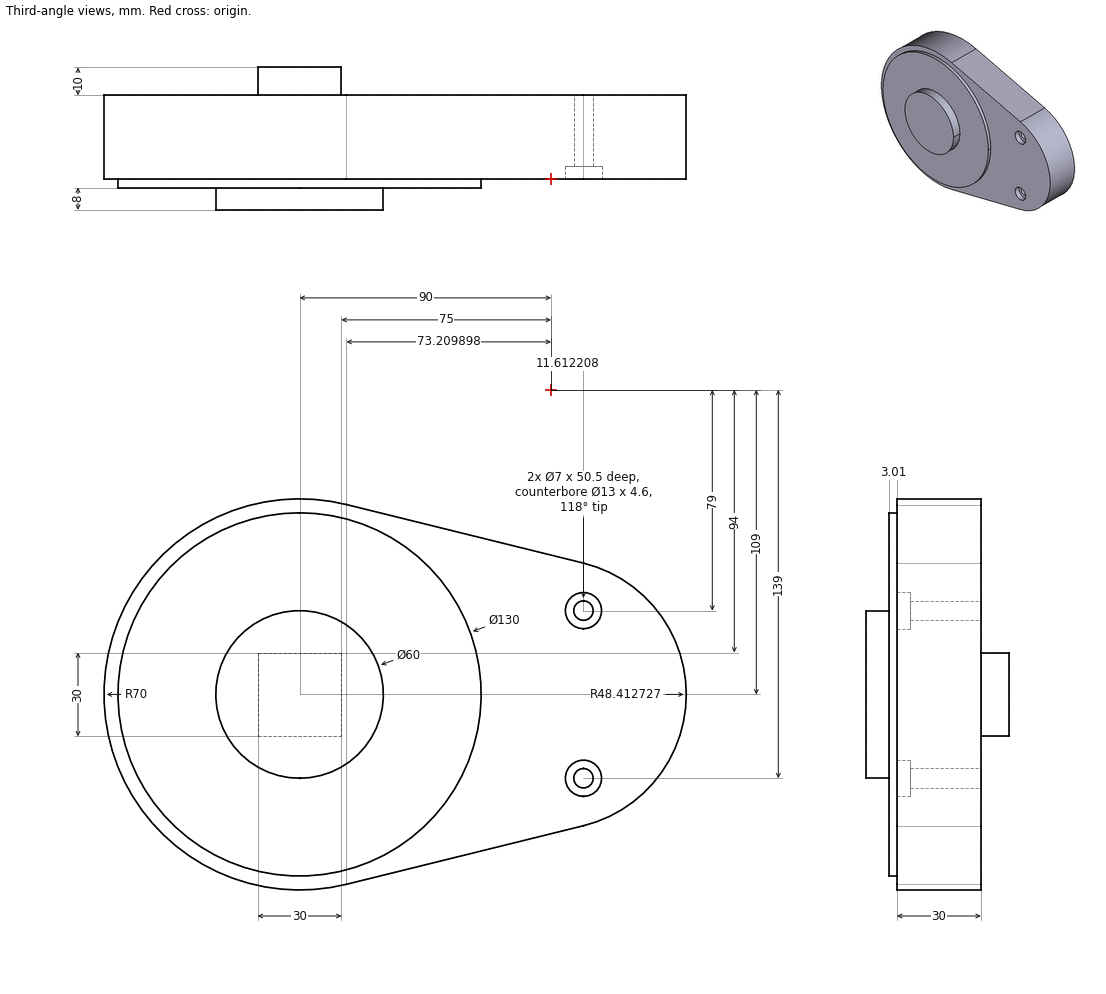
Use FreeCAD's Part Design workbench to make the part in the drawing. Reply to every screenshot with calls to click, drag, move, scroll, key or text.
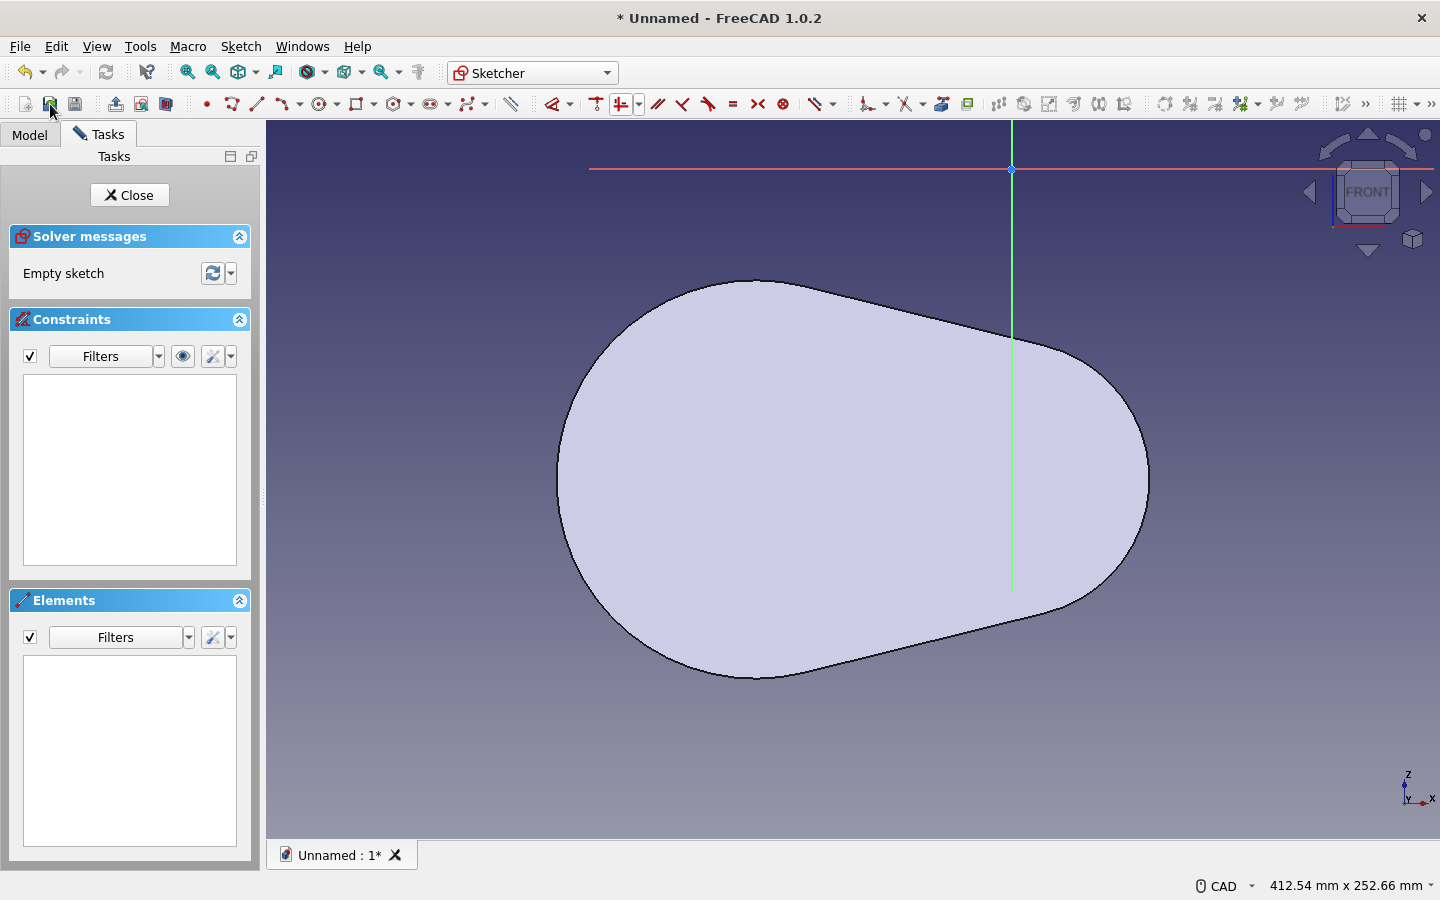
scroll(754, 762, down, 1)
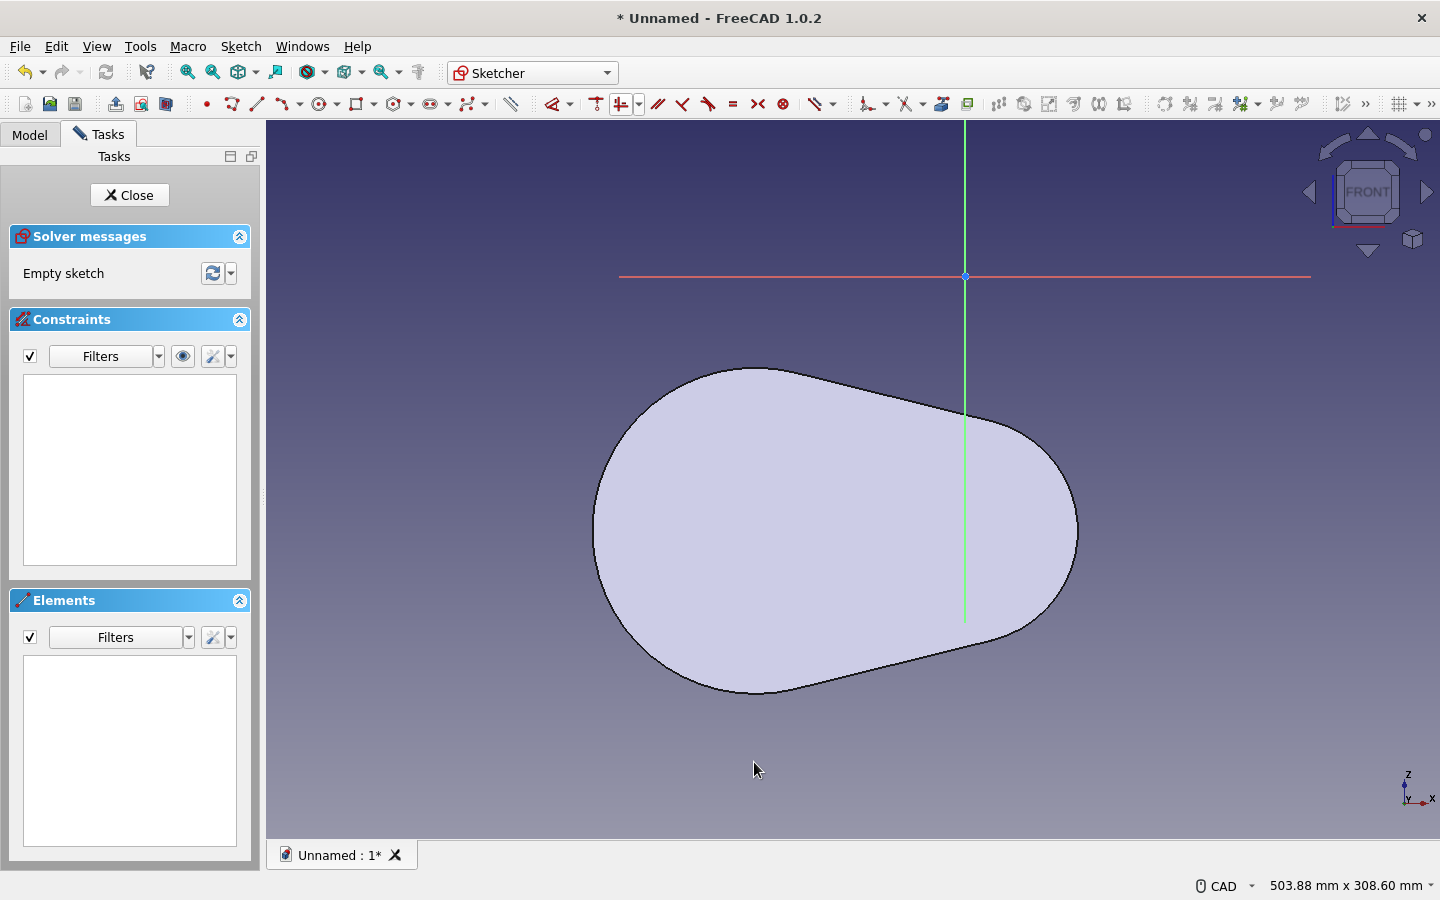
key(g)
key(c)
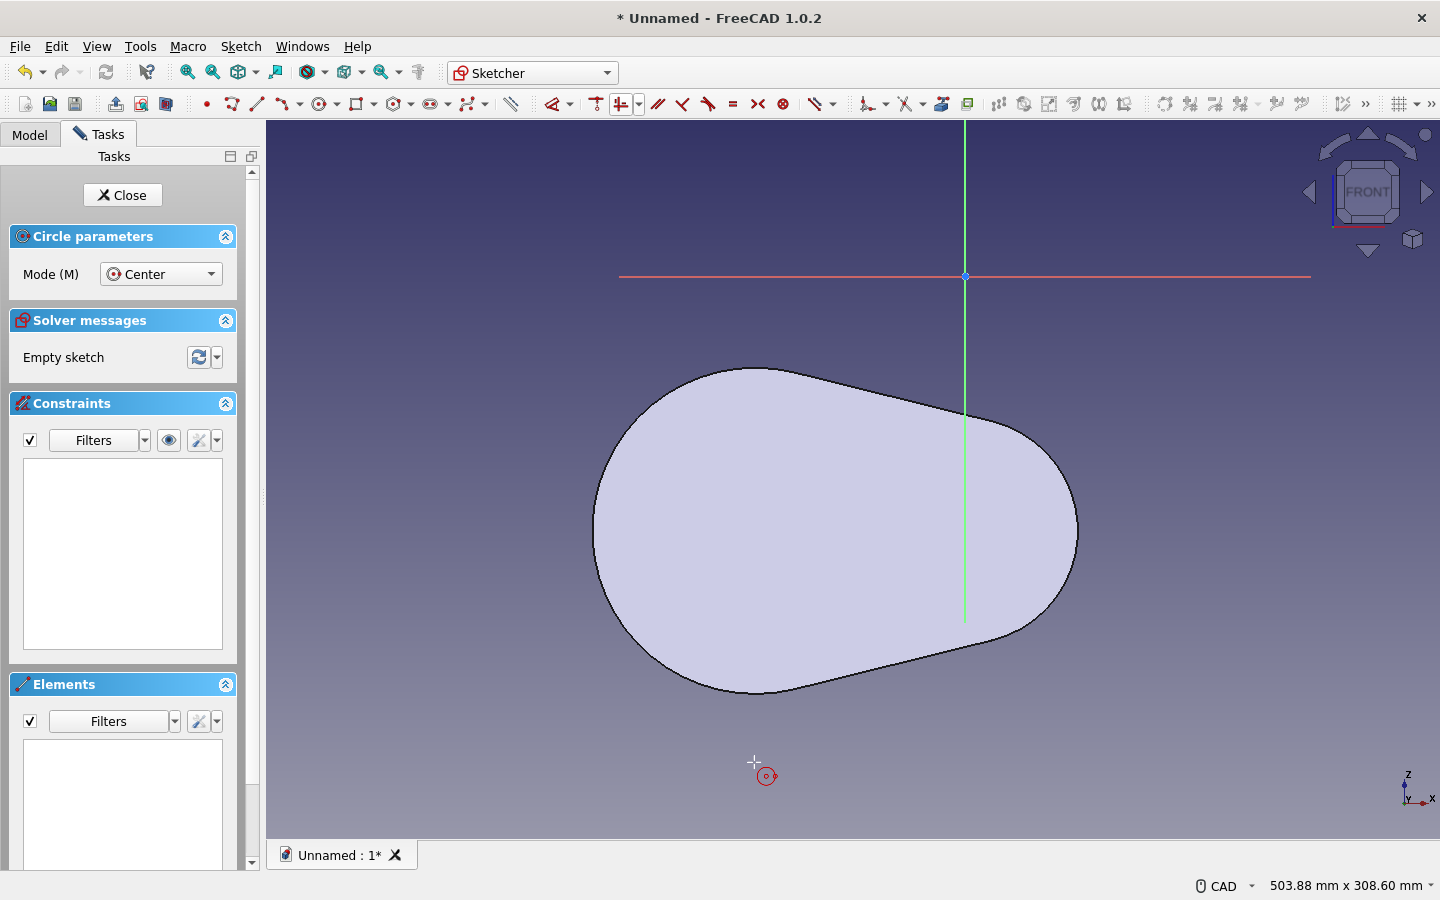
click(755, 531)
click(863, 424)
key(Escape)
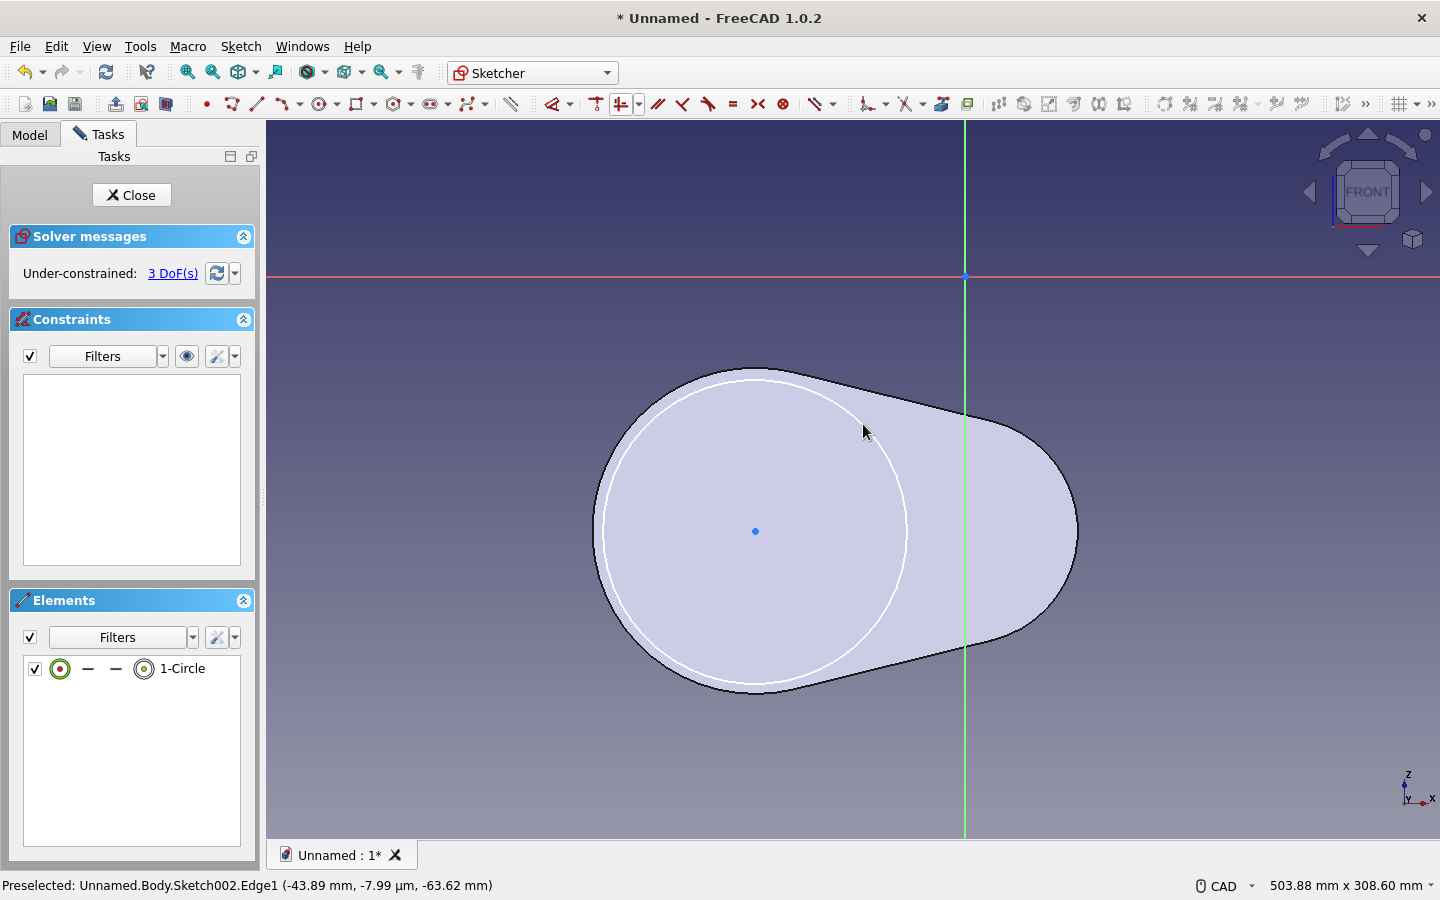
key(d)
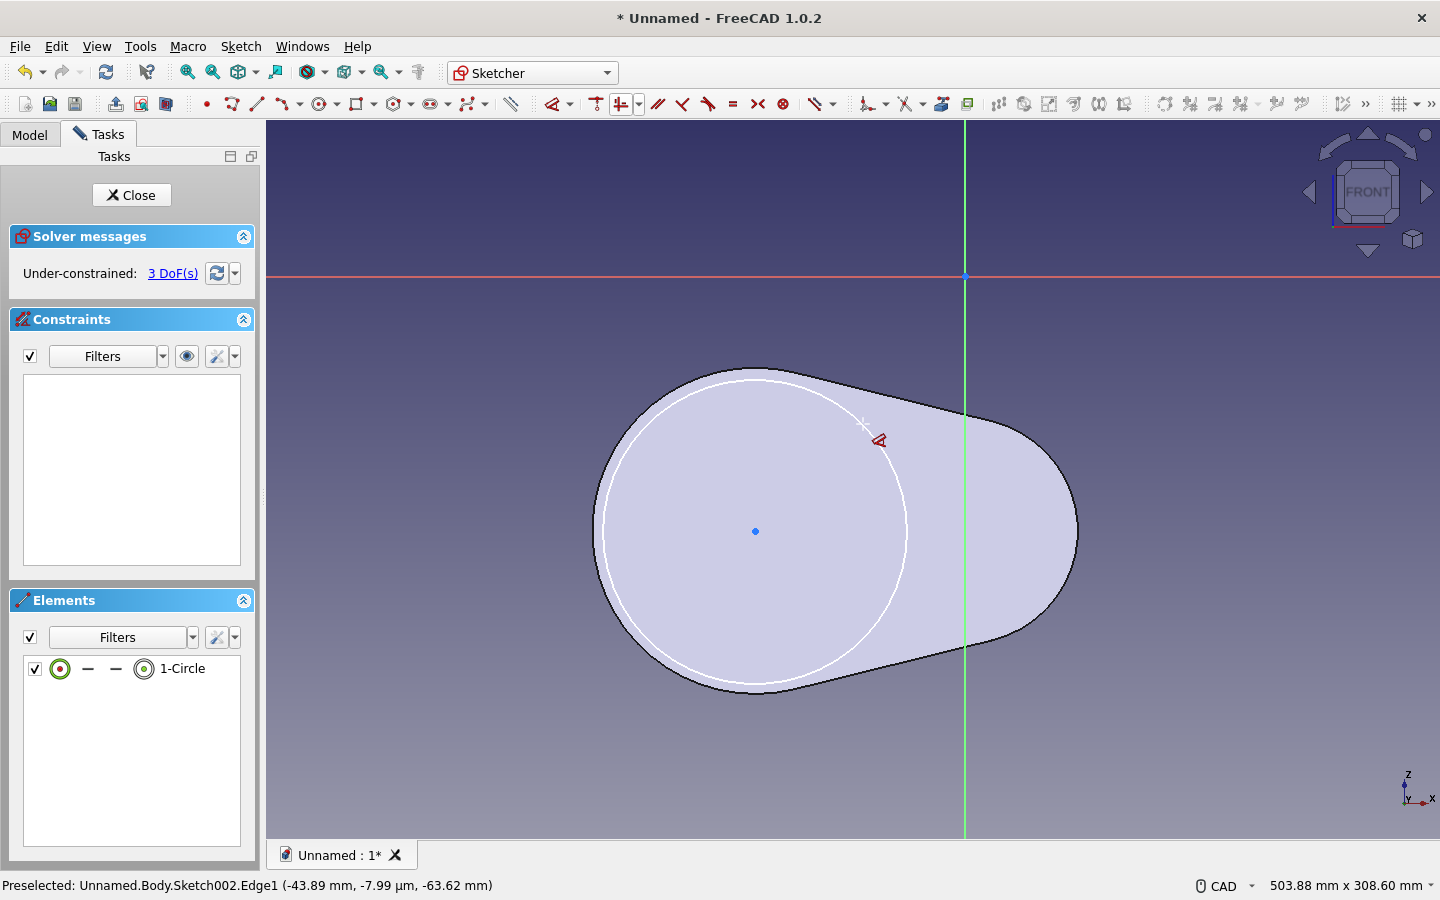
click(862, 424)
click(885, 401)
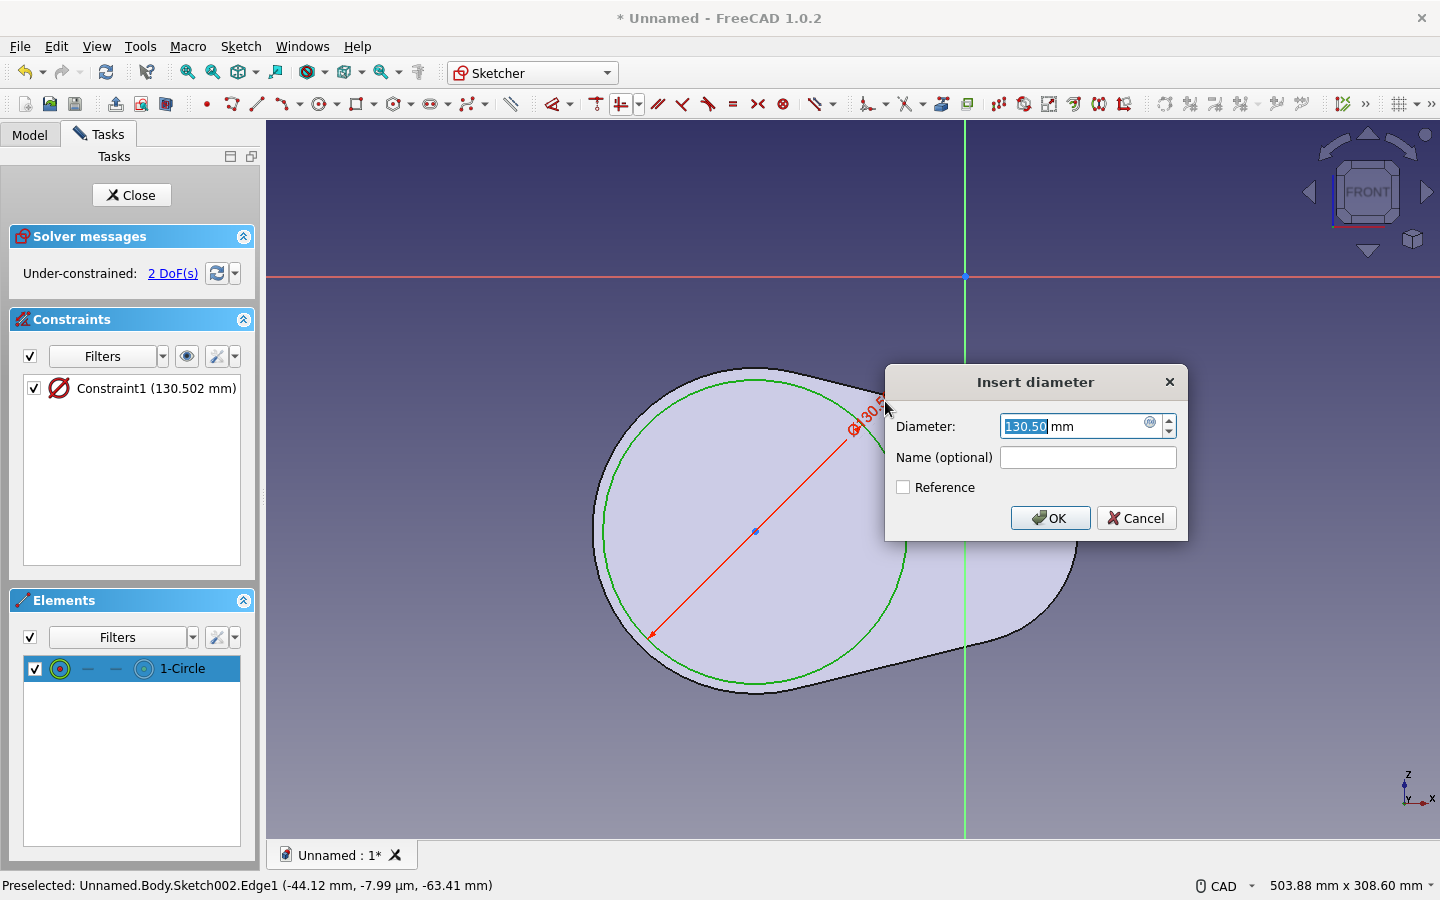
text(130)
key(Return)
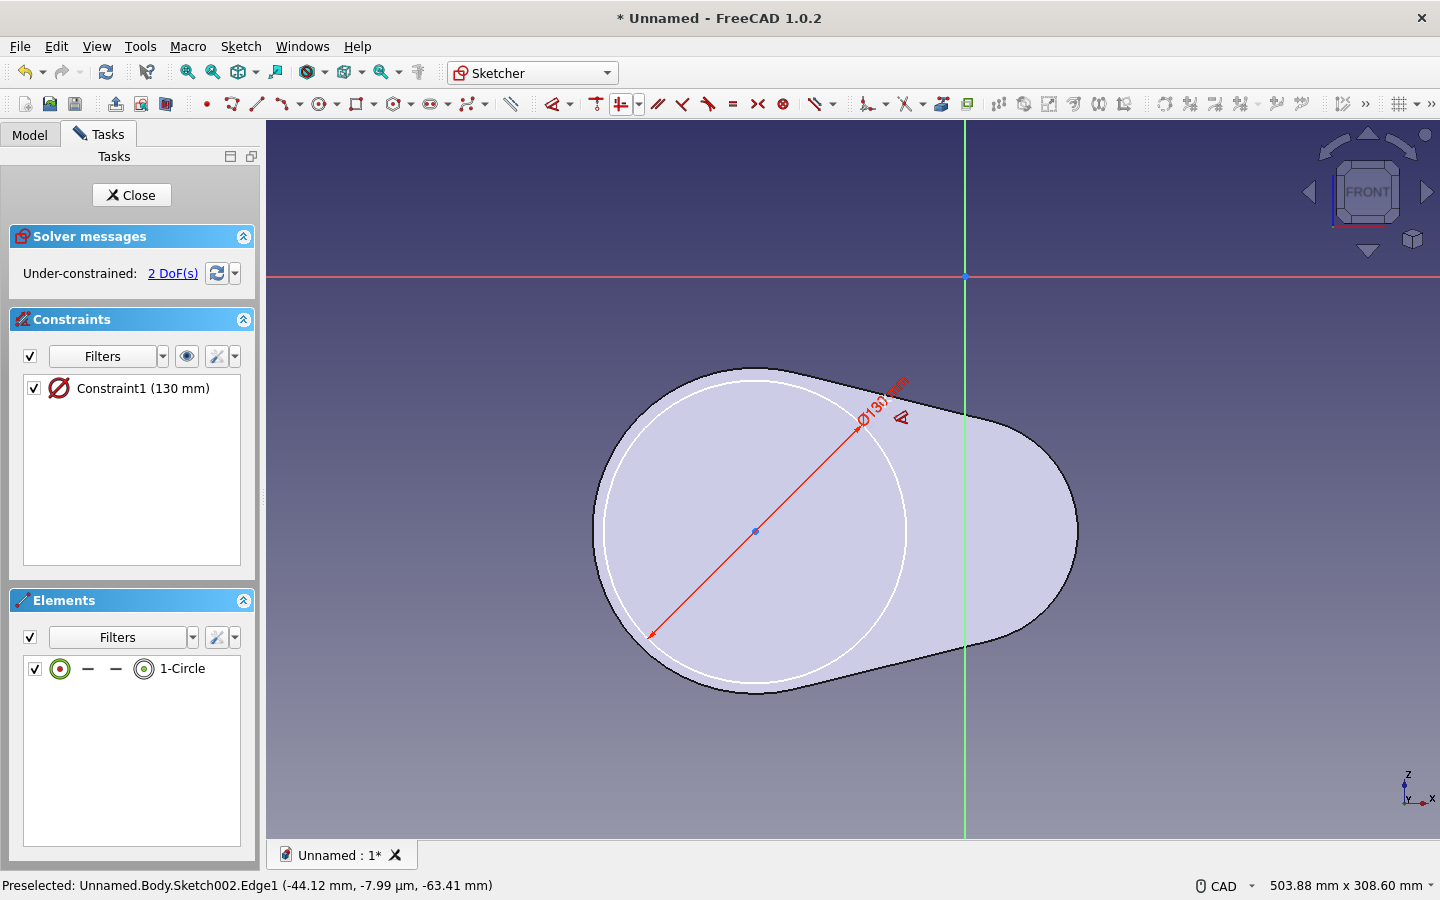
click(755, 532)
click(860, 243)